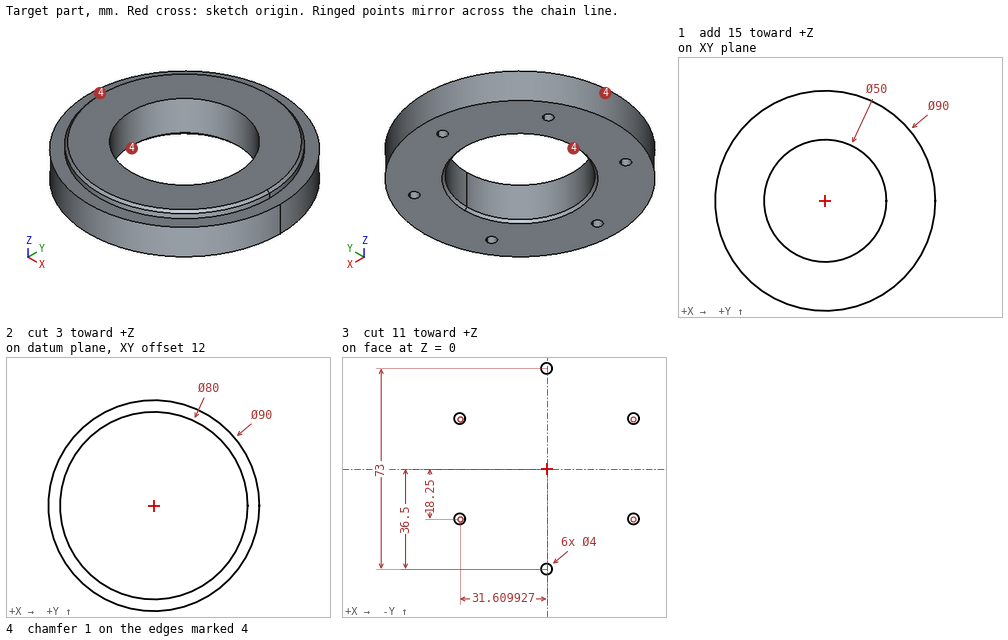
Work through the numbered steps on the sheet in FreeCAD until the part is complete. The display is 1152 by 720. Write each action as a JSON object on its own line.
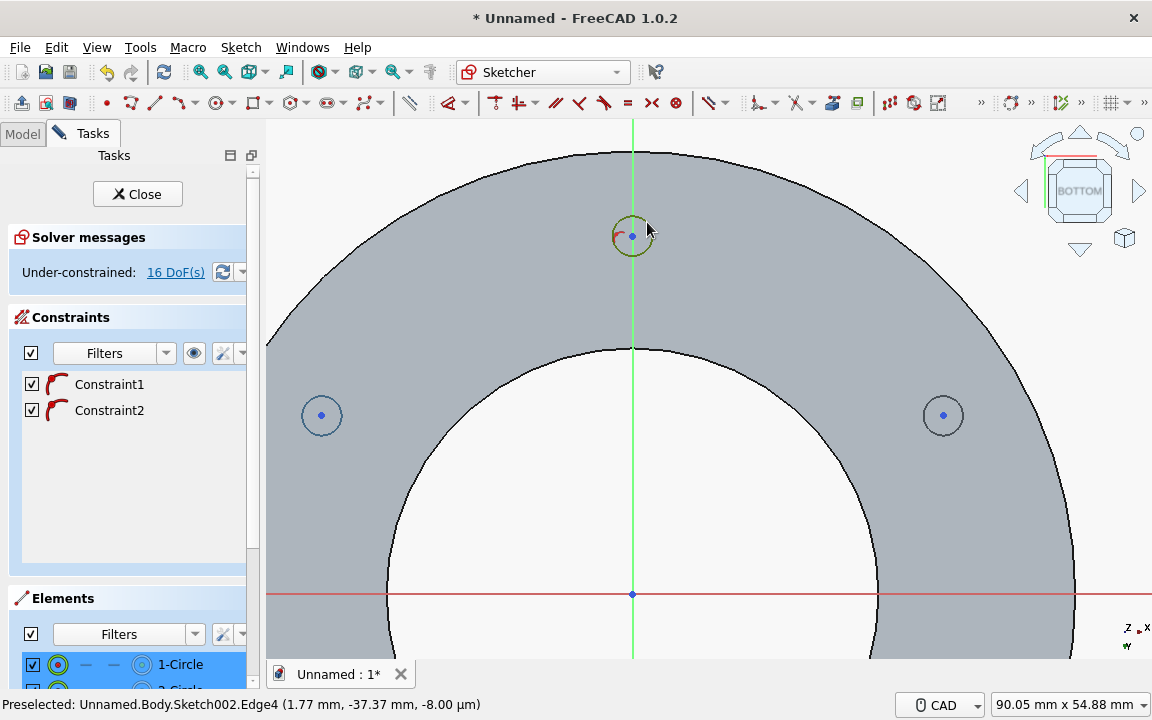
{"action": "left_click", "coordinate": [957, 402]}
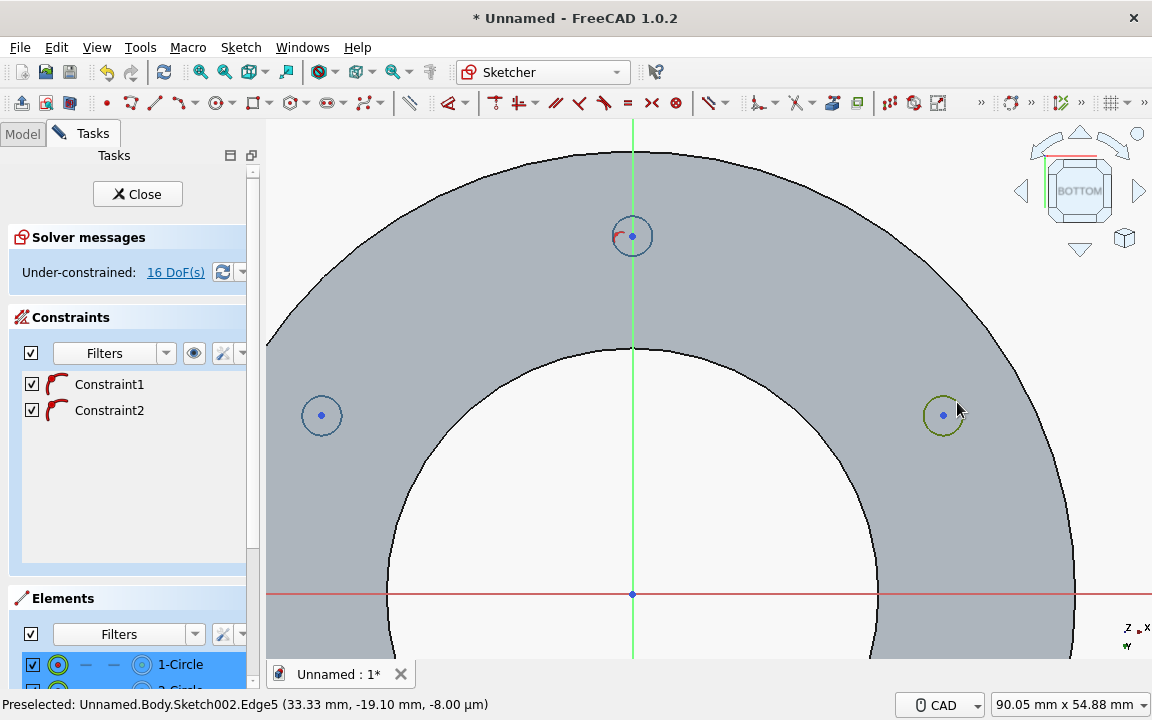
{"action": "scroll", "coordinate": [647, 221], "scroll_direction": "down", "scroll_amount": 4}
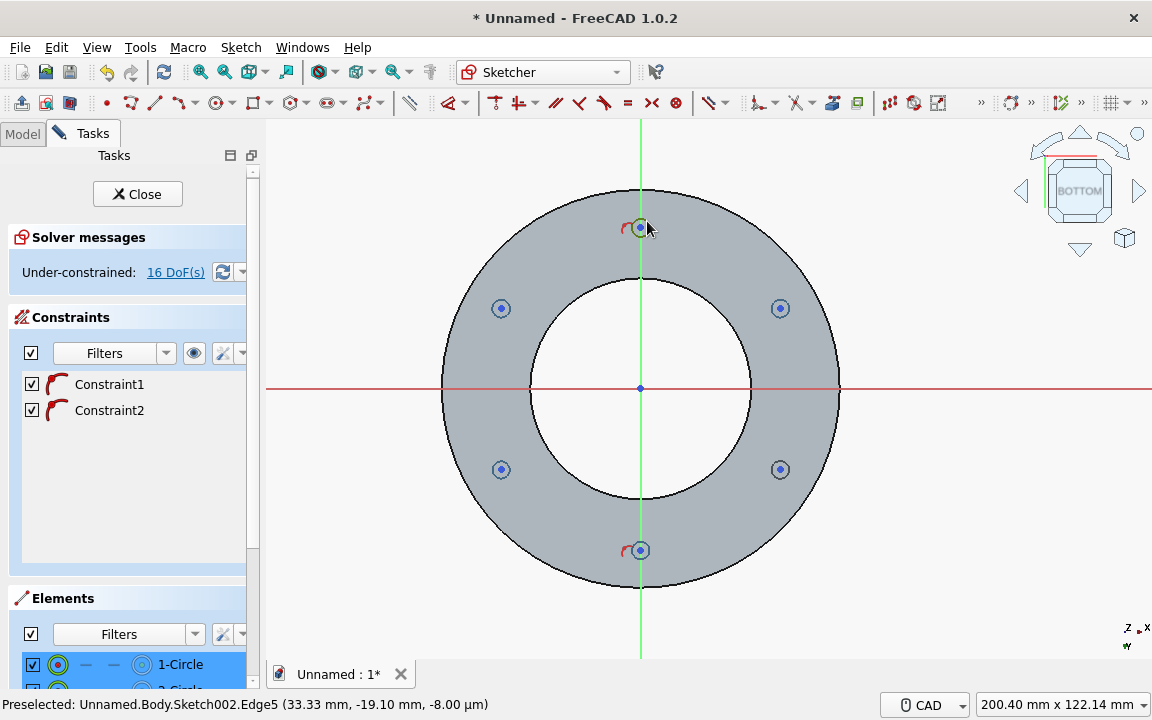
{"action": "scroll", "coordinate": [787, 464], "scroll_direction": "up", "scroll_amount": 3}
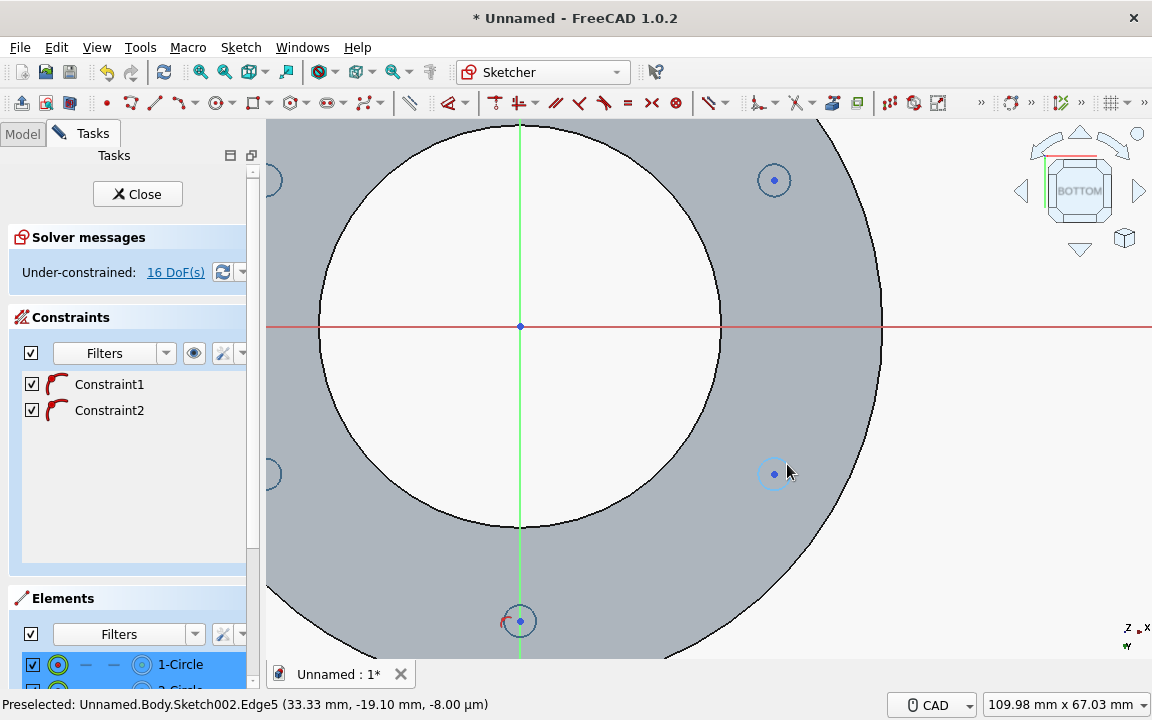
{"action": "left_click", "coordinate": [786, 463]}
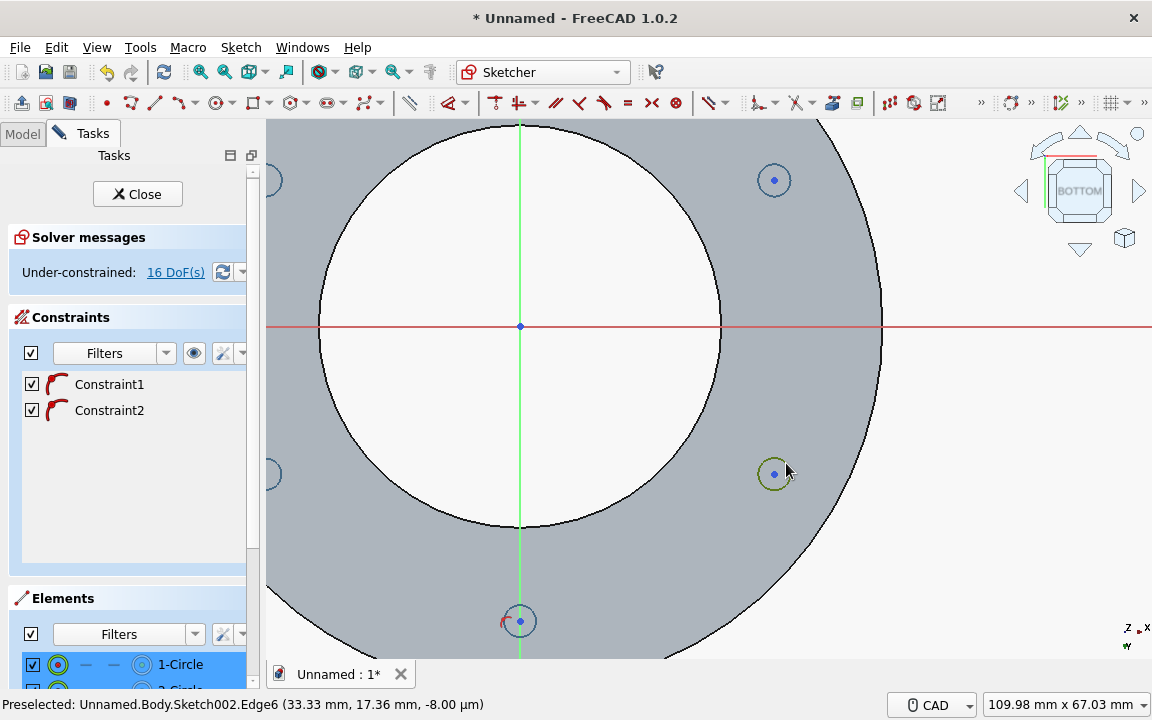
{"action": "key", "text": "e"}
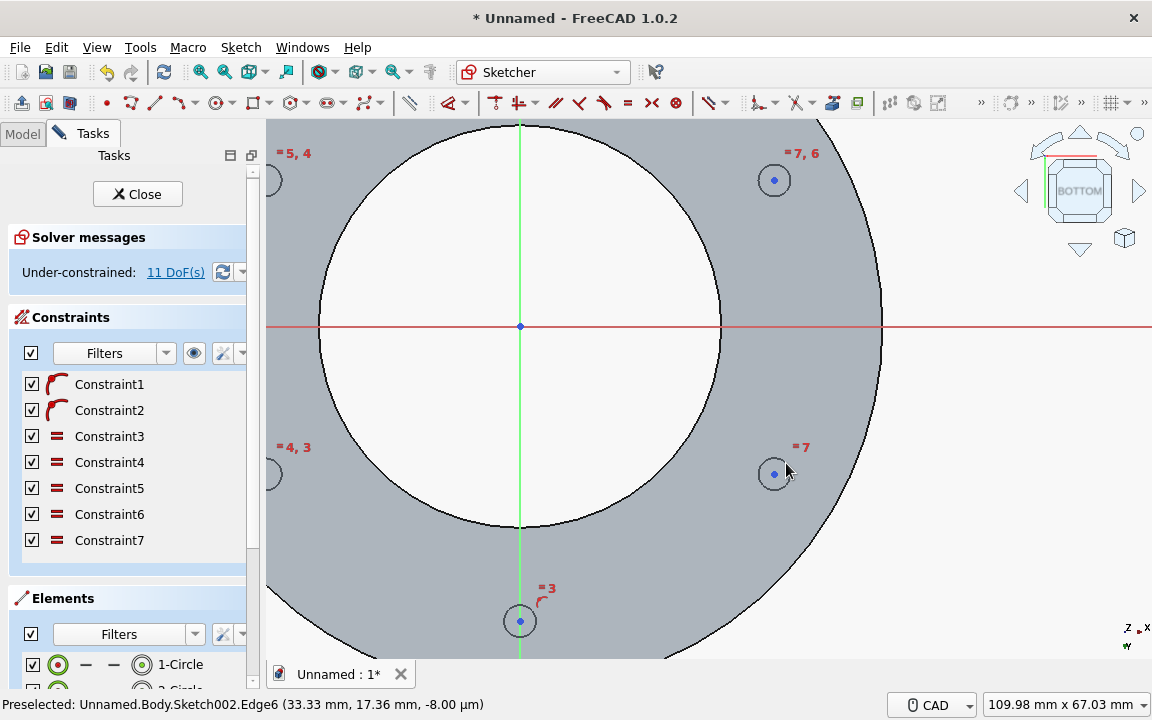
{"action": "scroll", "coordinate": [787, 465], "scroll_direction": "down", "scroll_amount": 3}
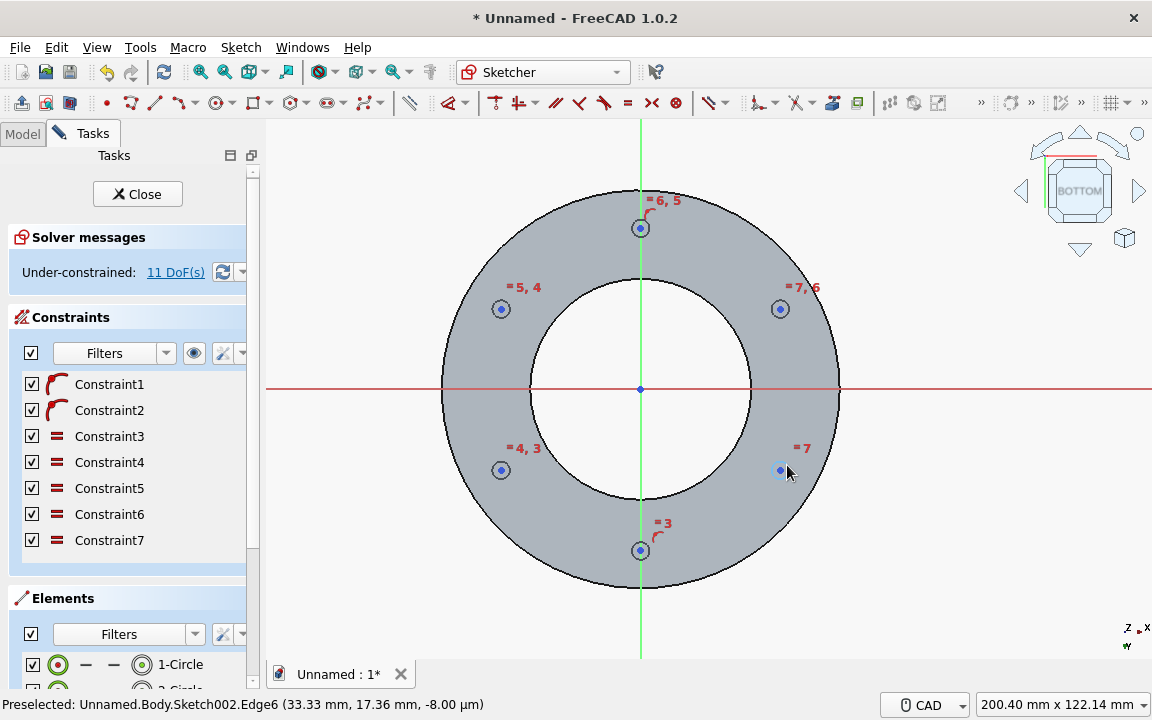
{"action": "left_click", "coordinate": [501, 470]}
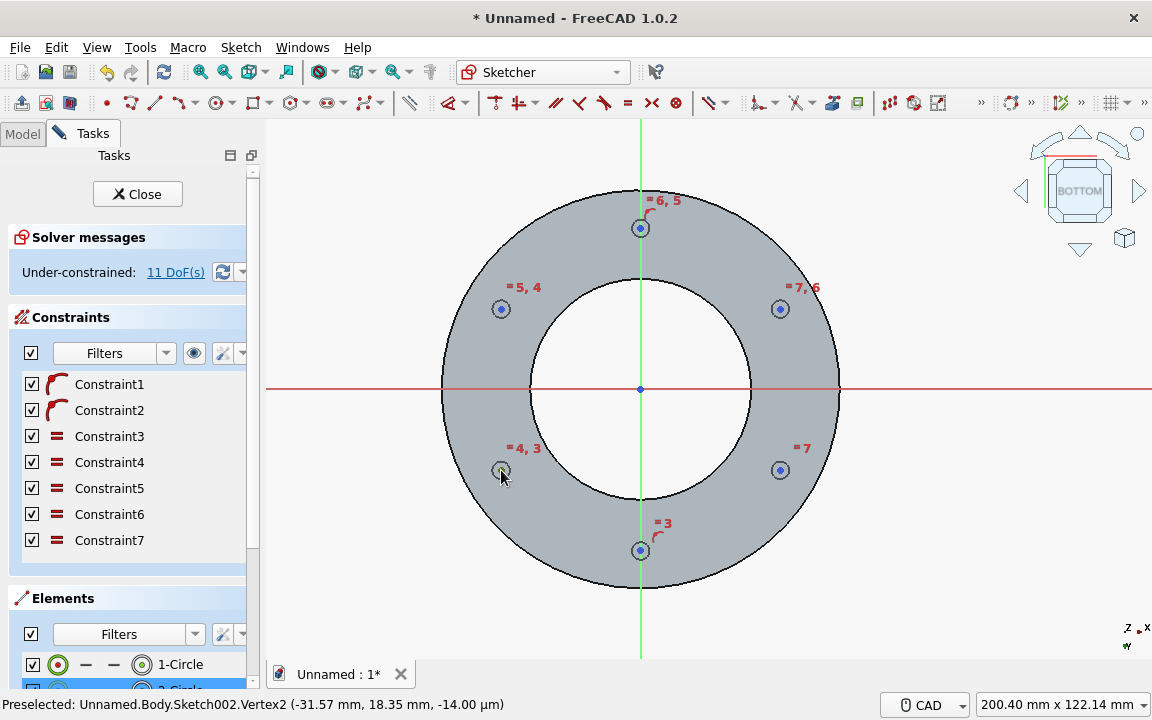
{"action": "left_click", "coordinate": [501, 309]}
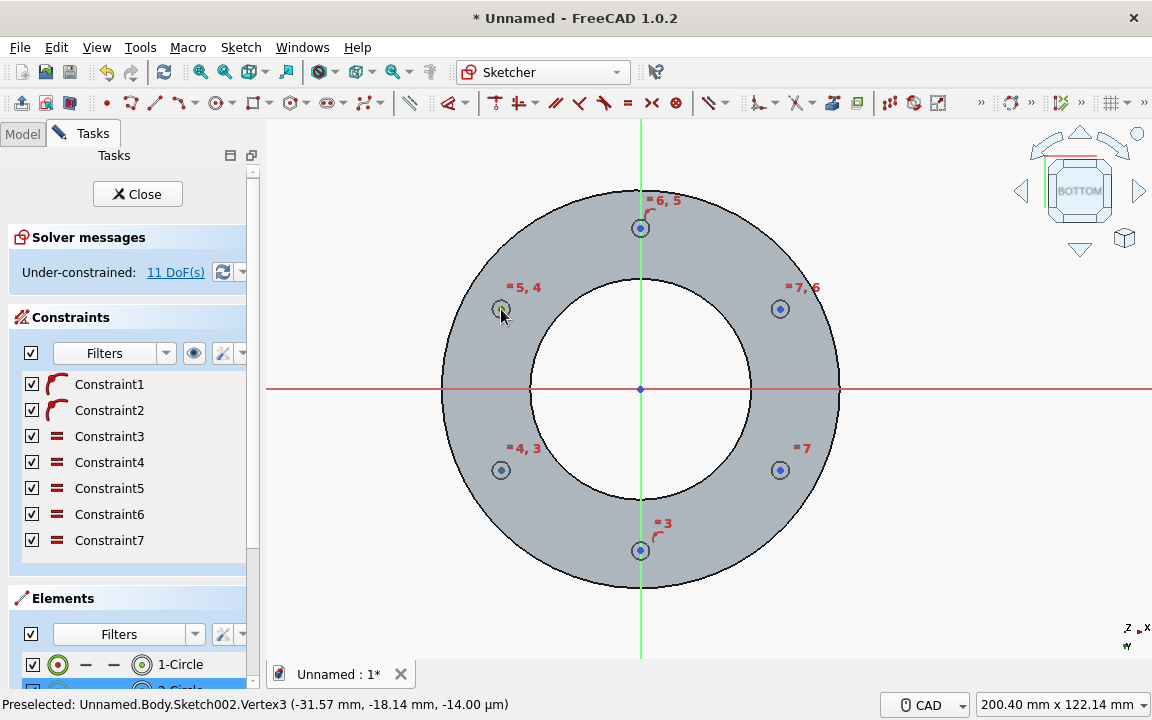
{"action": "left_click", "coordinate": [344, 389]}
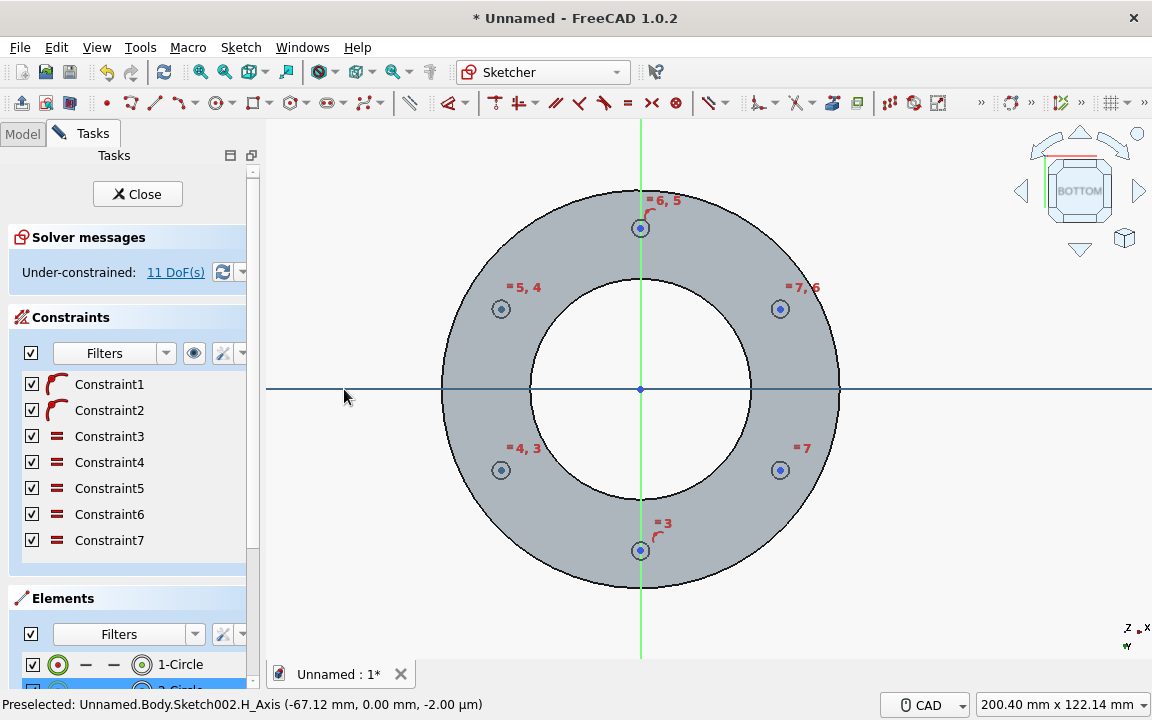
{"action": "left_click", "coordinate": [652, 104]}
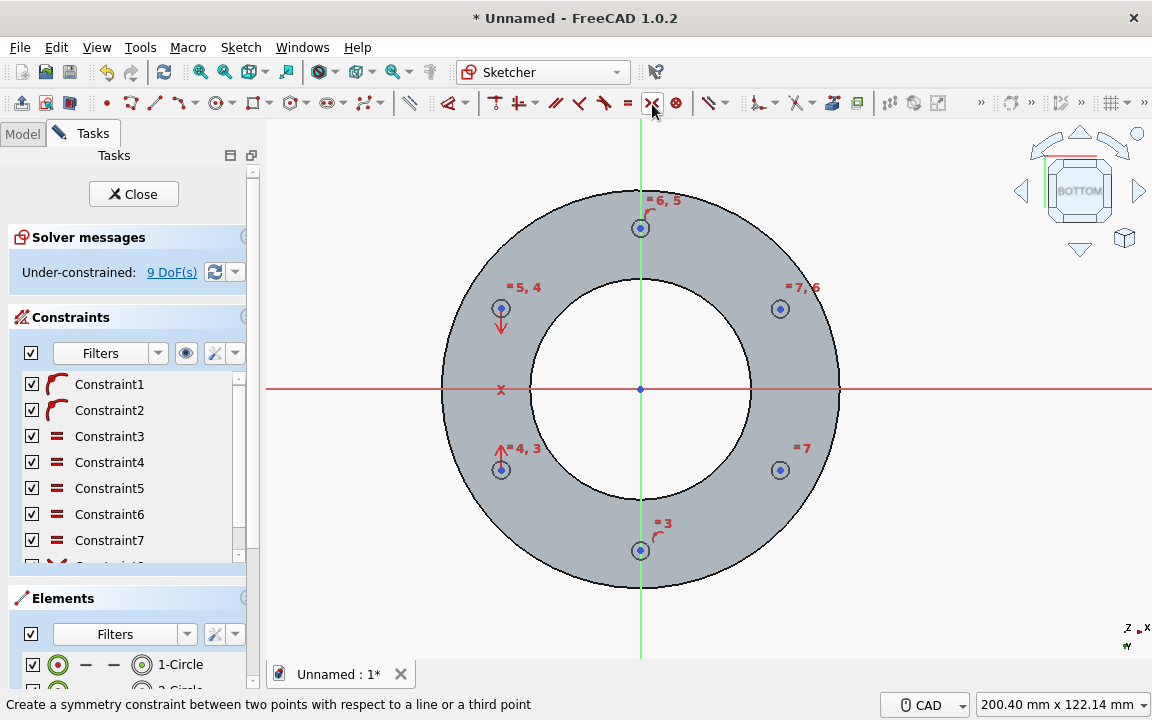
{"action": "left_click", "coordinate": [501, 309]}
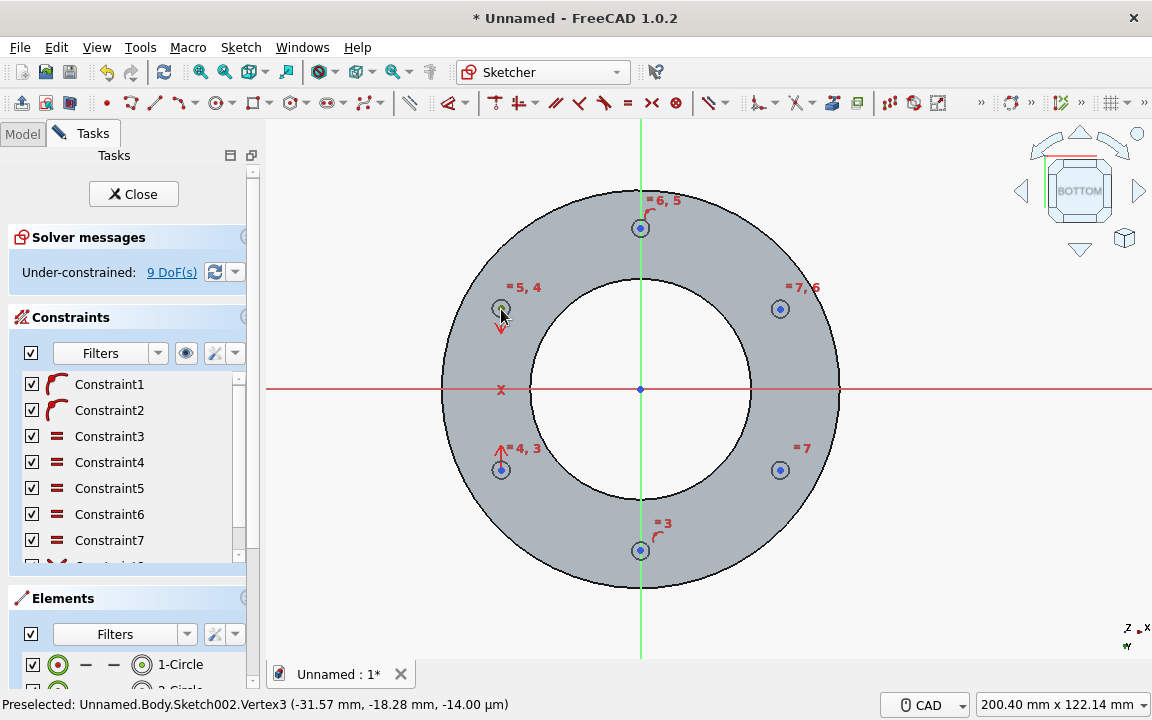
{"action": "left_click", "coordinate": [780, 309]}